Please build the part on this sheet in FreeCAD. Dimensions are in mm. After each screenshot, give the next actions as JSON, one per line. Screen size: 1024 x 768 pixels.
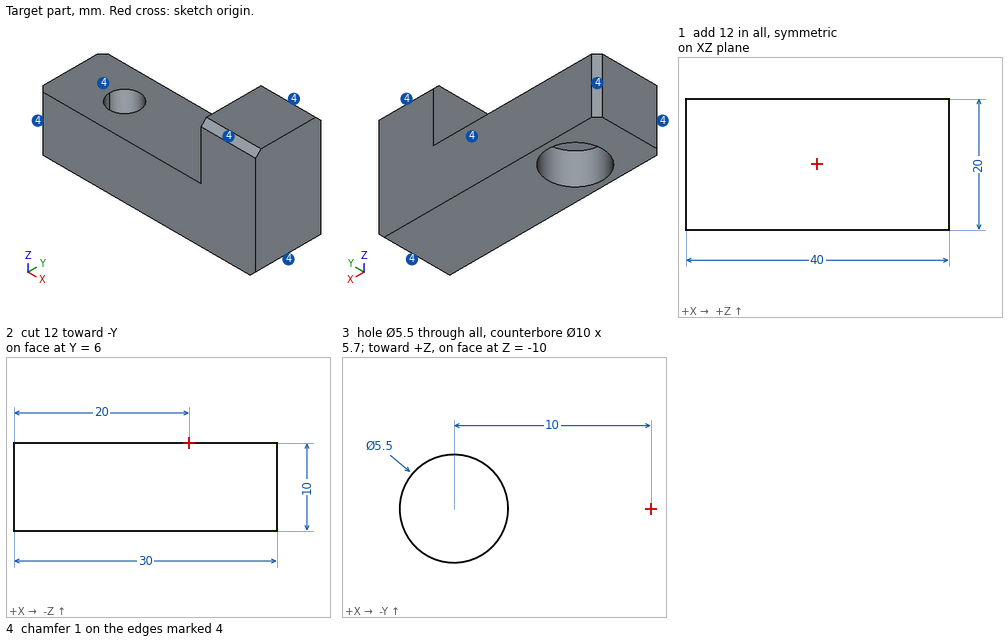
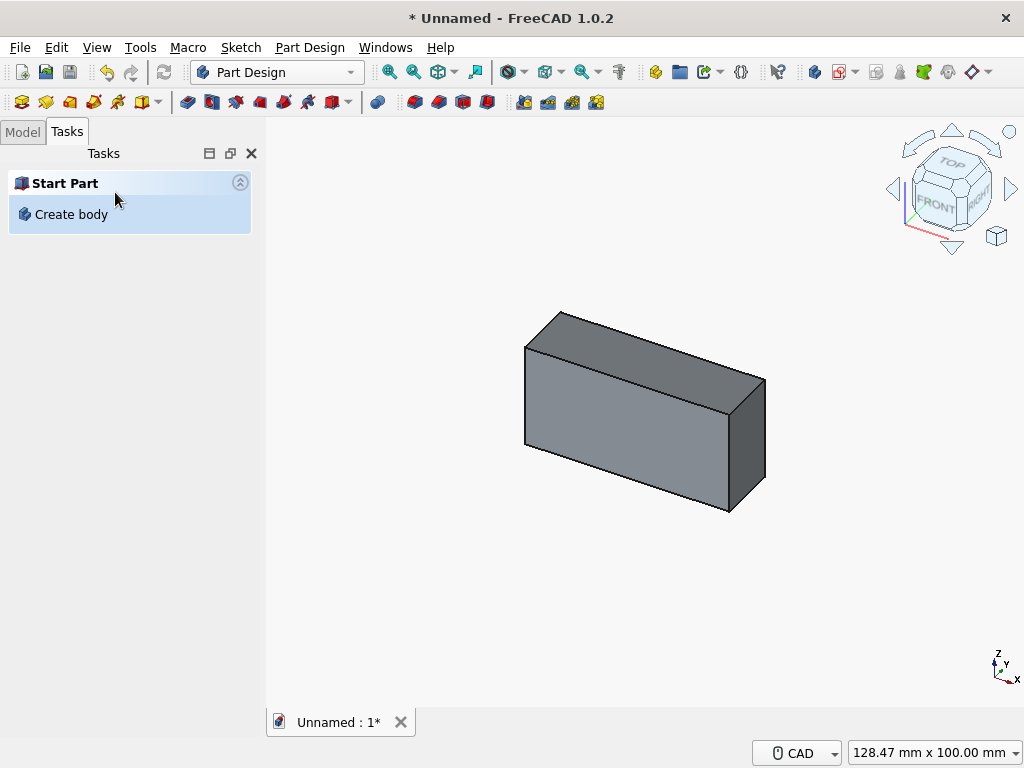
{"action": "key", "text": "v f"}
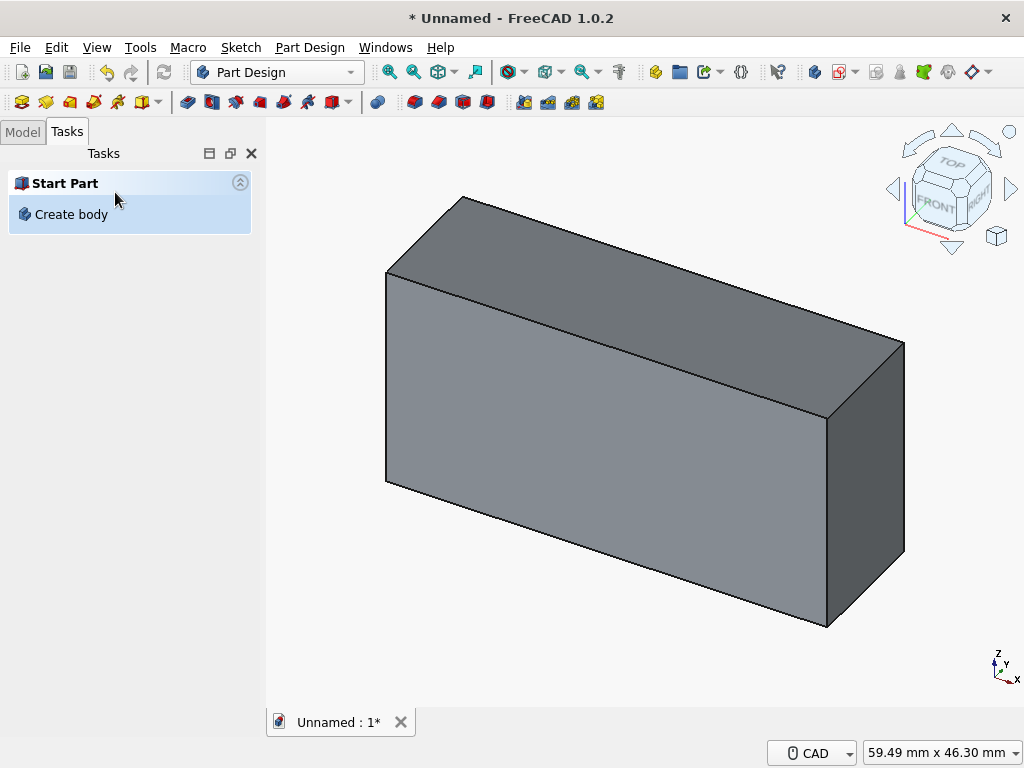
{"action": "key", "text": "4"}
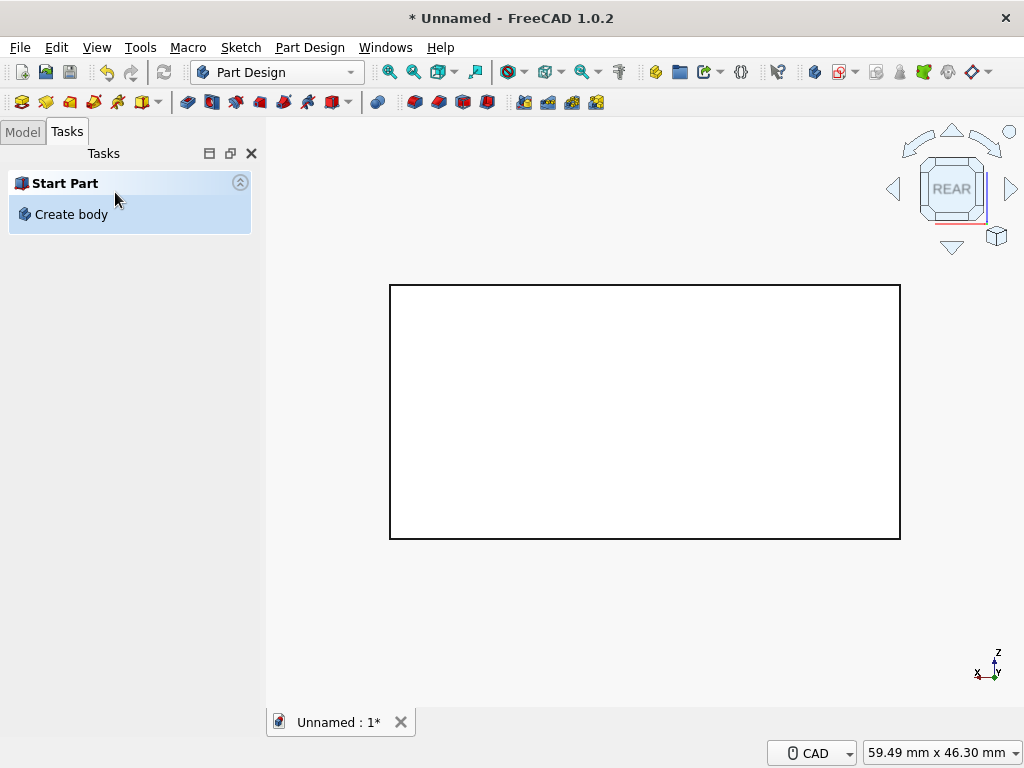
{"action": "left_click", "coordinate": [572, 411]}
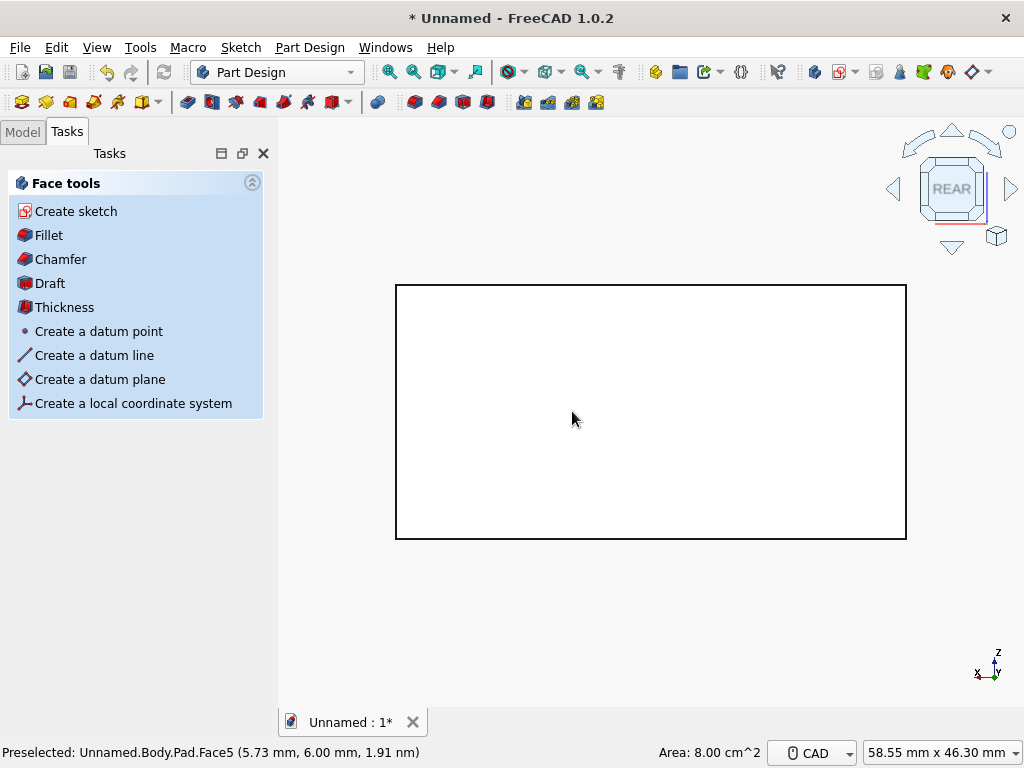
{"action": "left_click", "coordinate": [840, 72]}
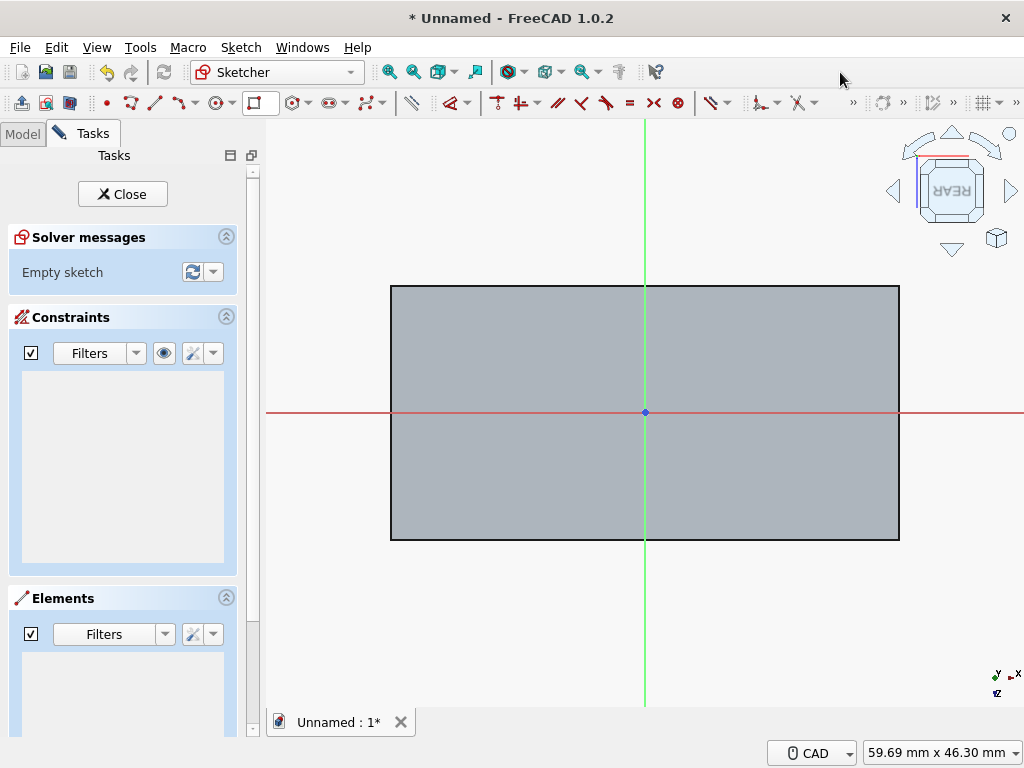
{"action": "key", "text": "g r"}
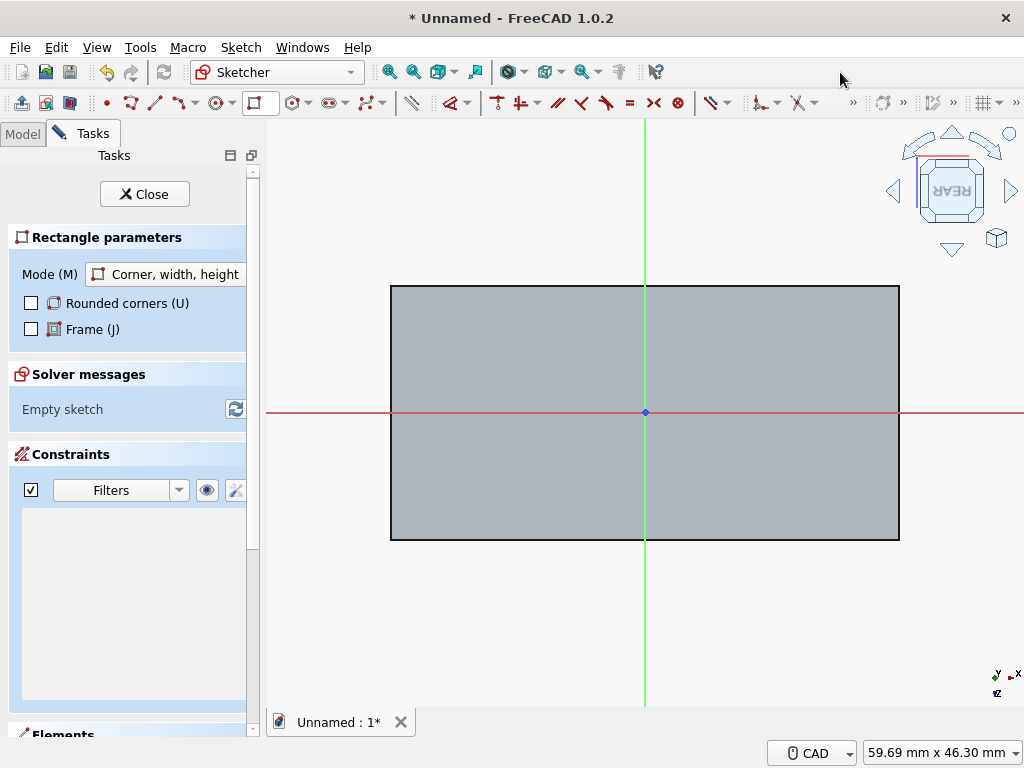
{"action": "left_click", "coordinate": [391, 413]}
{"action": "mouse_move", "coordinate": [772, 540]}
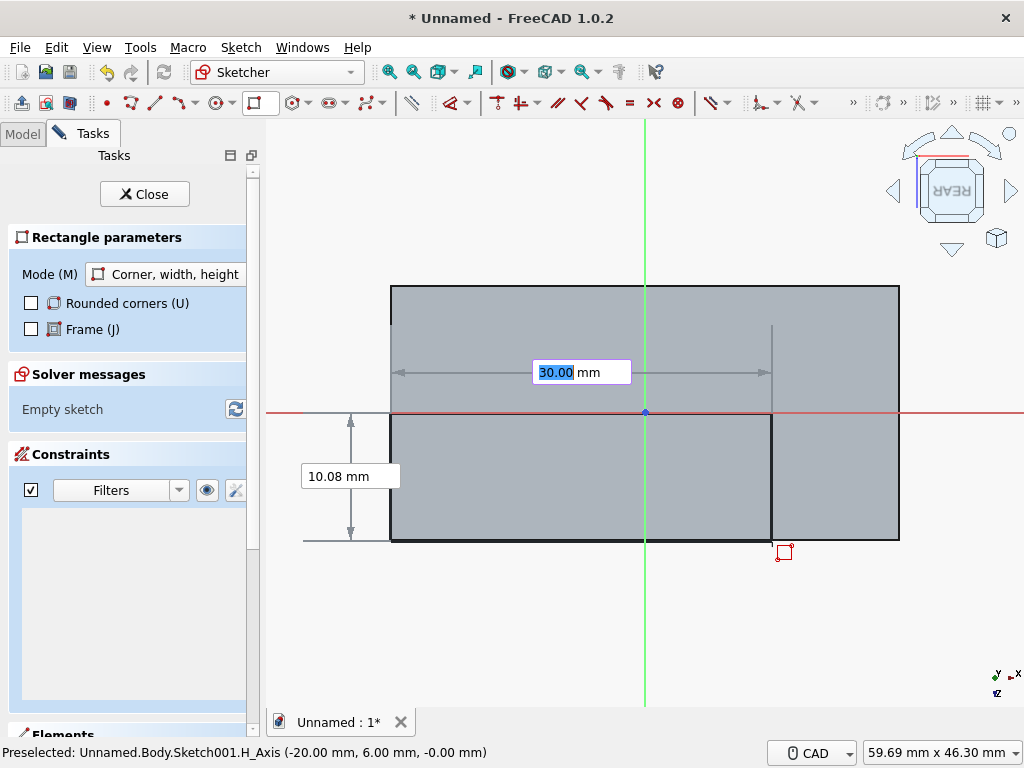
{"action": "type", "text": "30"}
{"action": "key", "text": "Tab"}
{"action": "type", "text": "10"}
{"action": "key", "text": "Return"}
{"action": "key", "text": "Escape"}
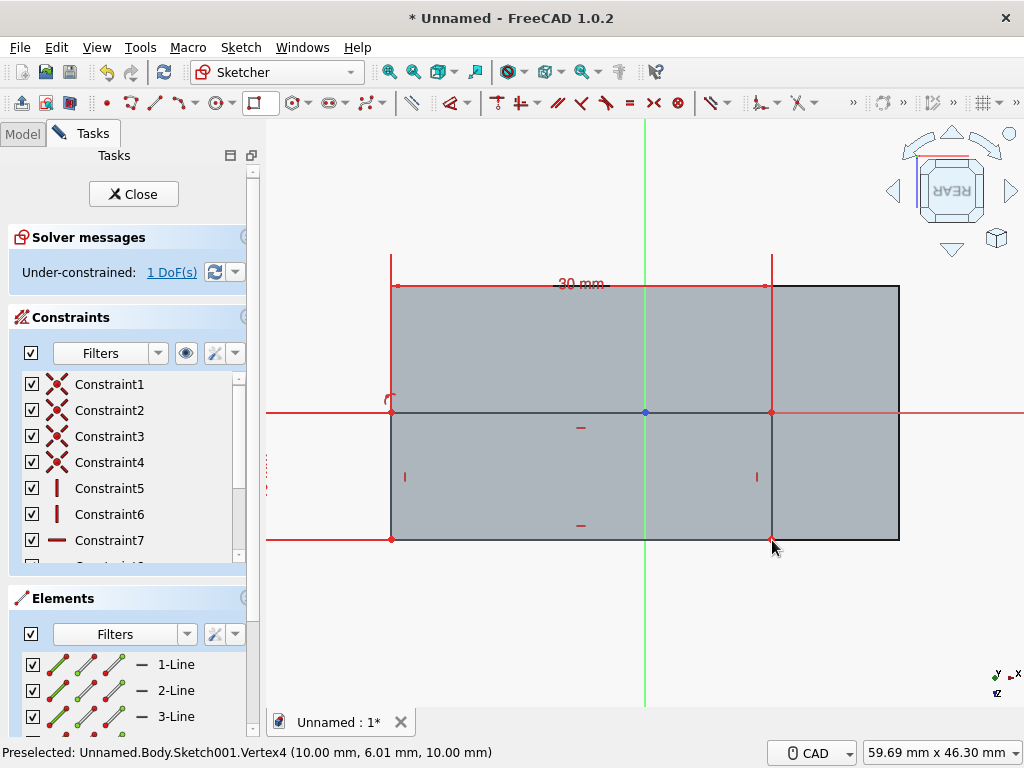
{"action": "left_click", "coordinate": [391, 413]}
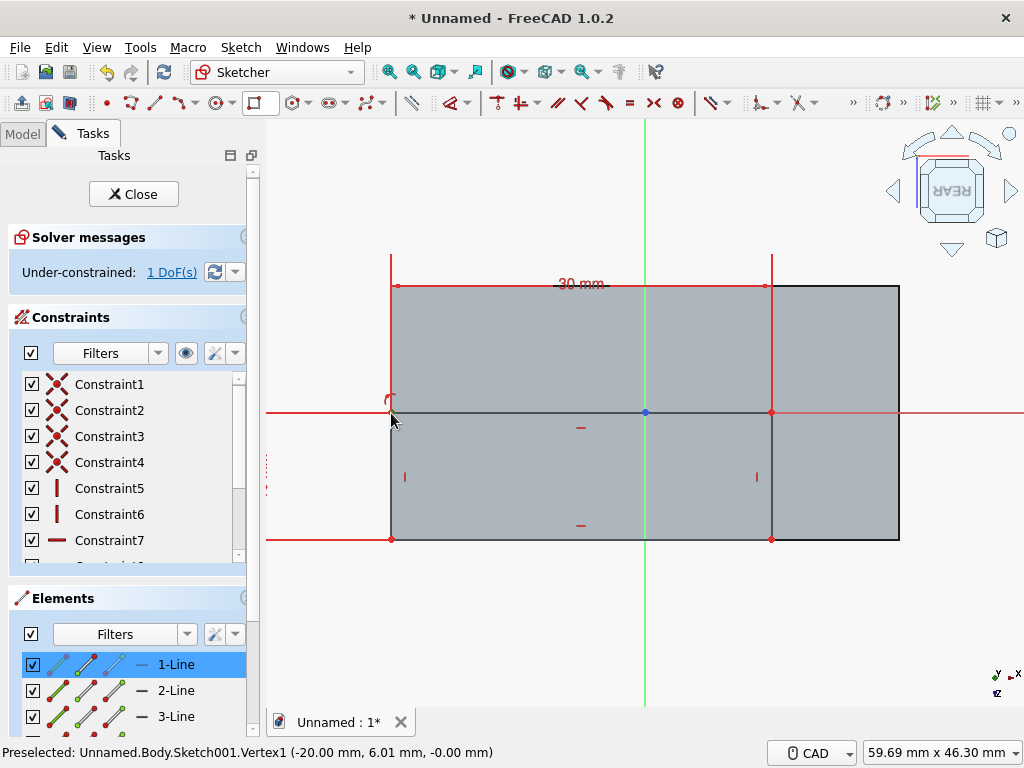
{"action": "key", "text": "l"}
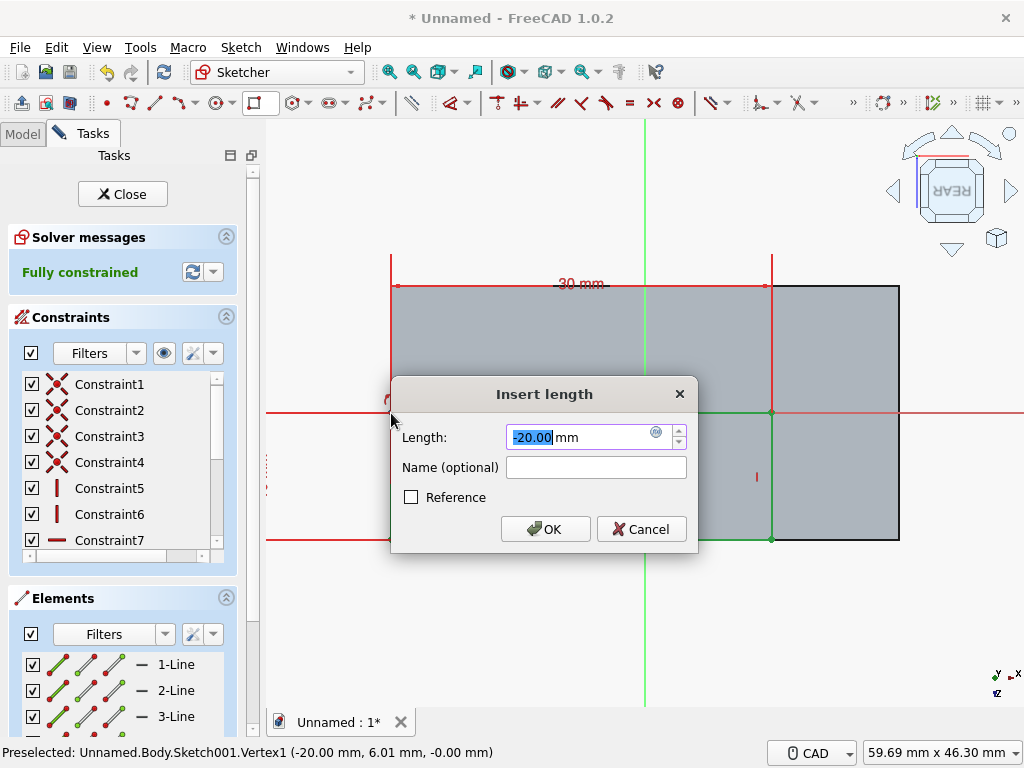
{"action": "type", "text": "-20"}
{"action": "key", "text": "Return"}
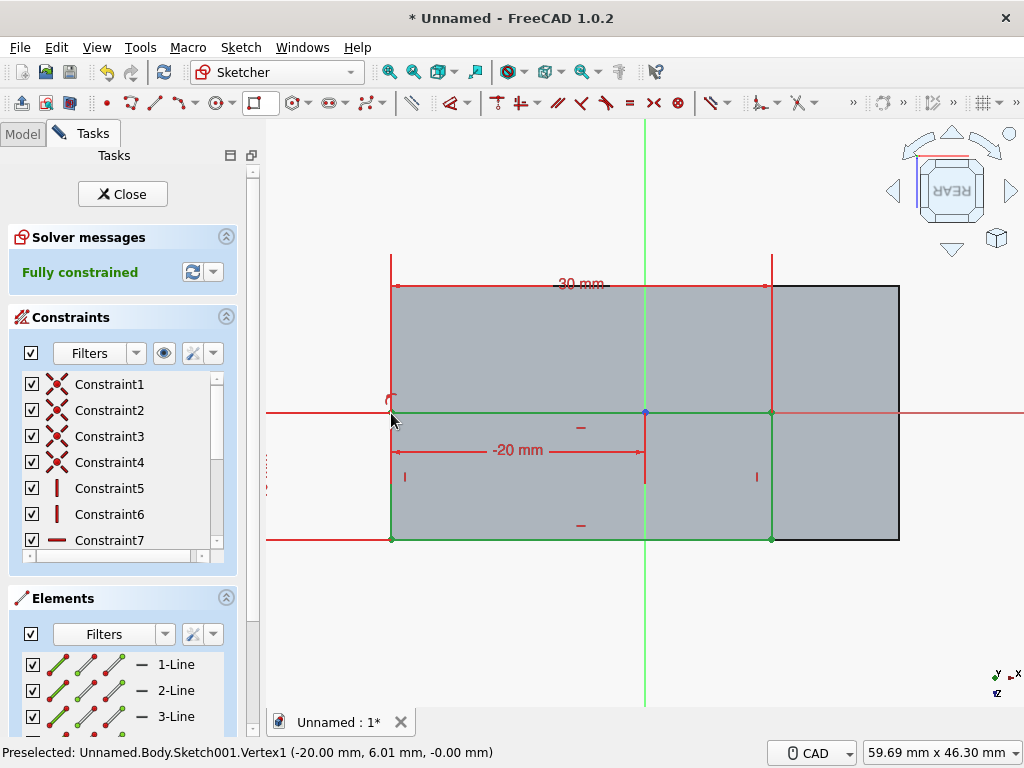
{"action": "left_click", "coordinate": [123, 194]}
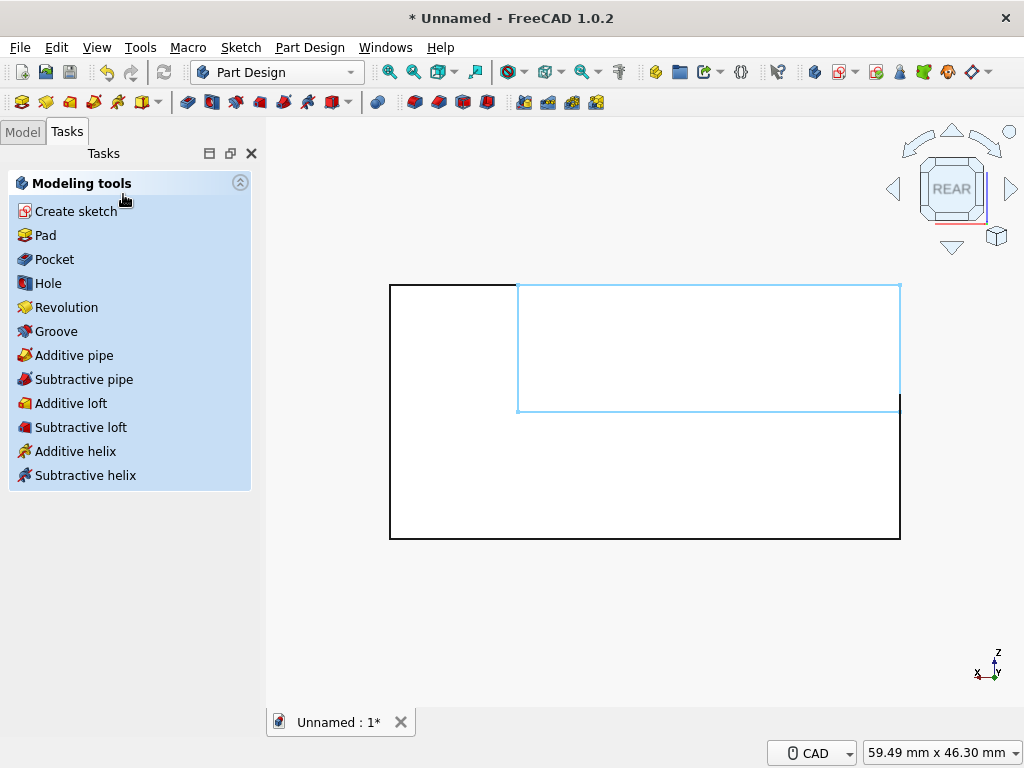
{"action": "left_click", "coordinate": [188, 102]}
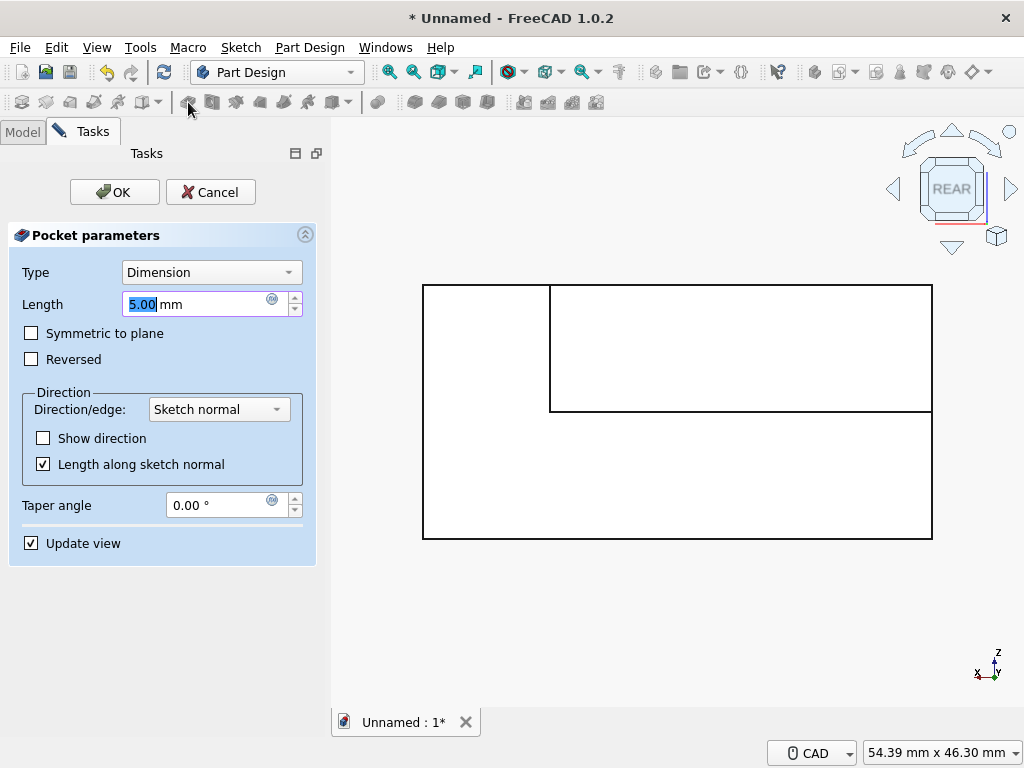
{"action": "type", "text": "12"}
{"action": "key", "text": "Tab"}